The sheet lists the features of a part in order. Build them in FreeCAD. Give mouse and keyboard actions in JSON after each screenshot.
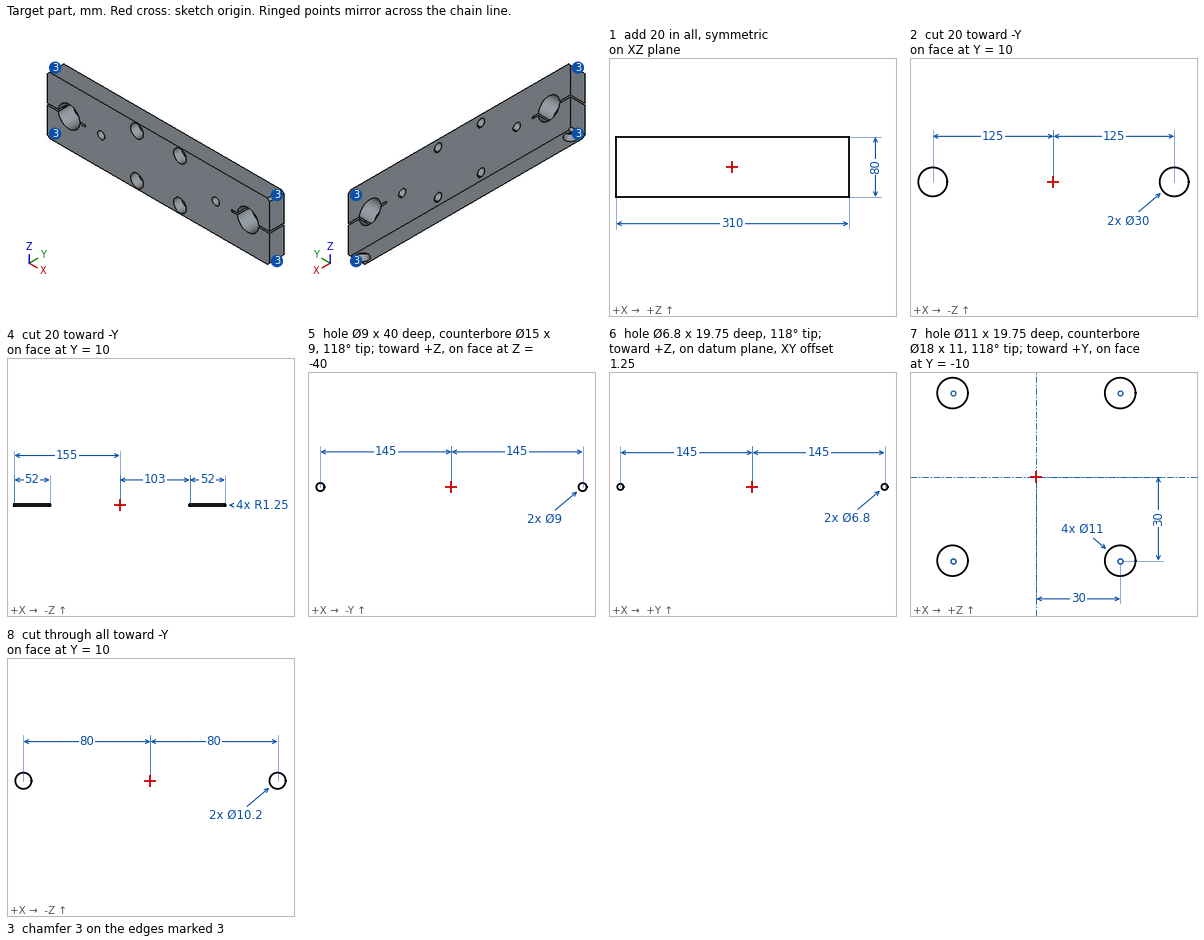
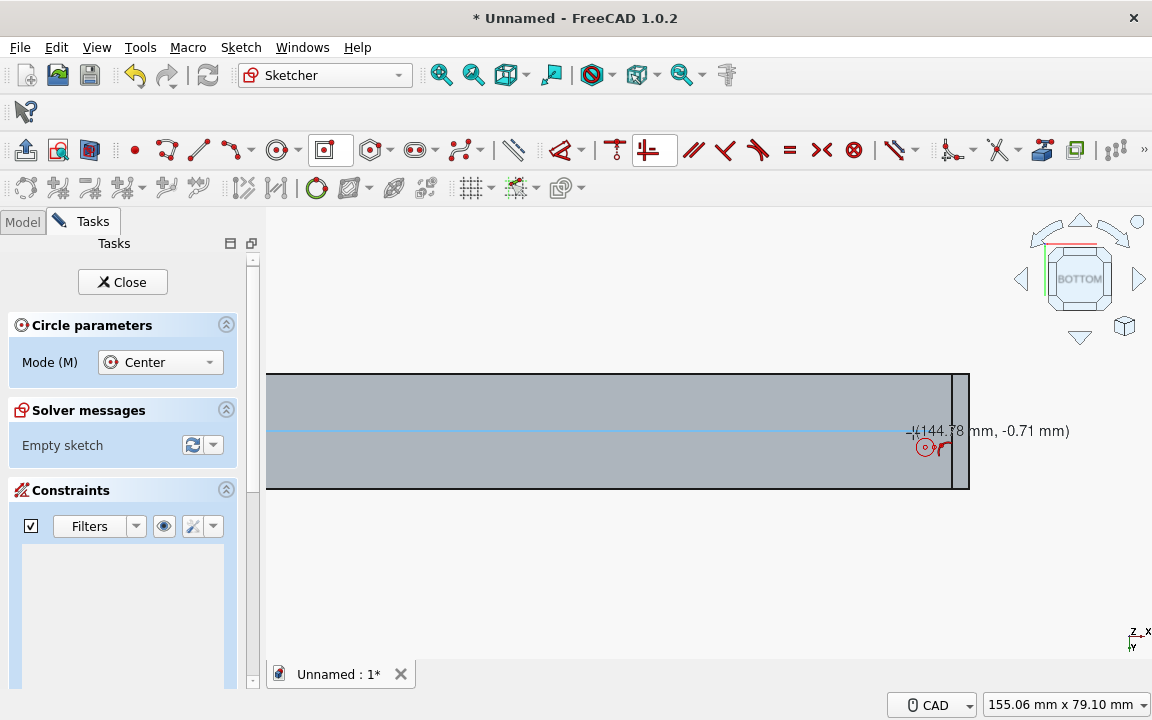
{"action": "scroll", "coordinate": [881, 434], "scroll_direction": "down", "scroll_amount": 6}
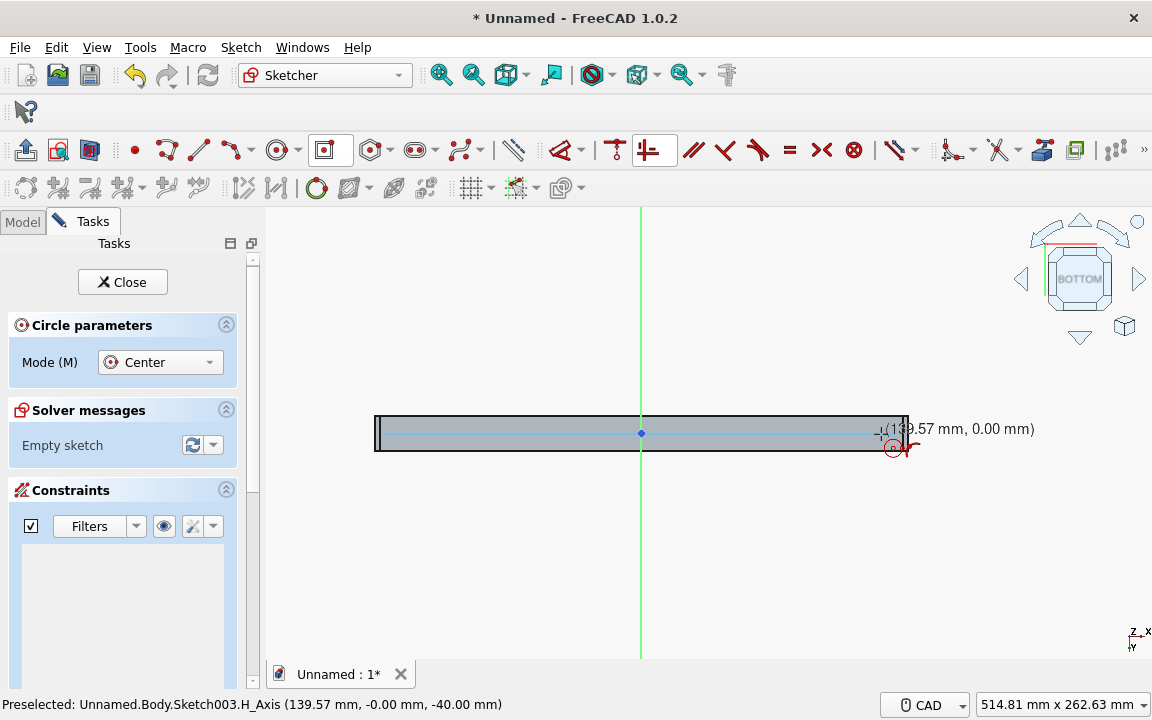
{"action": "left_click", "coordinate": [891, 434]}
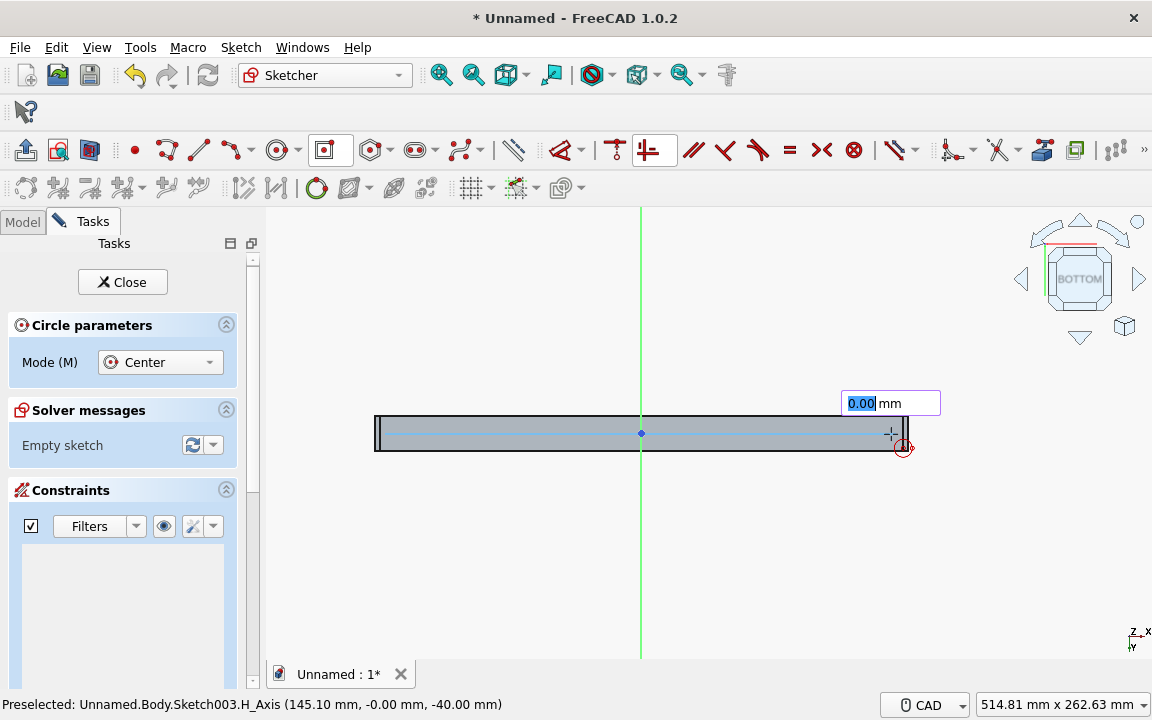
{"action": "scroll", "coordinate": [888, 441], "scroll_direction": "up", "scroll_amount": 4}
{"action": "mouse_move", "coordinate": [888, 440]}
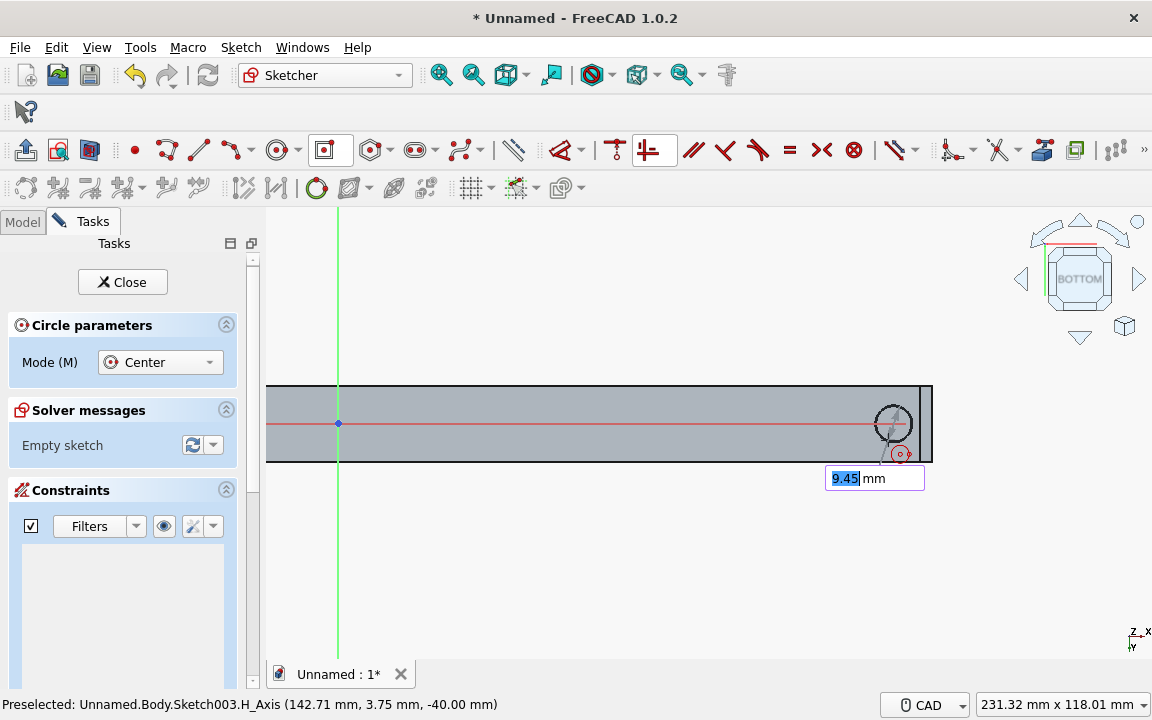
{"action": "type", "text": "9"}
{"action": "key", "text": "Return"}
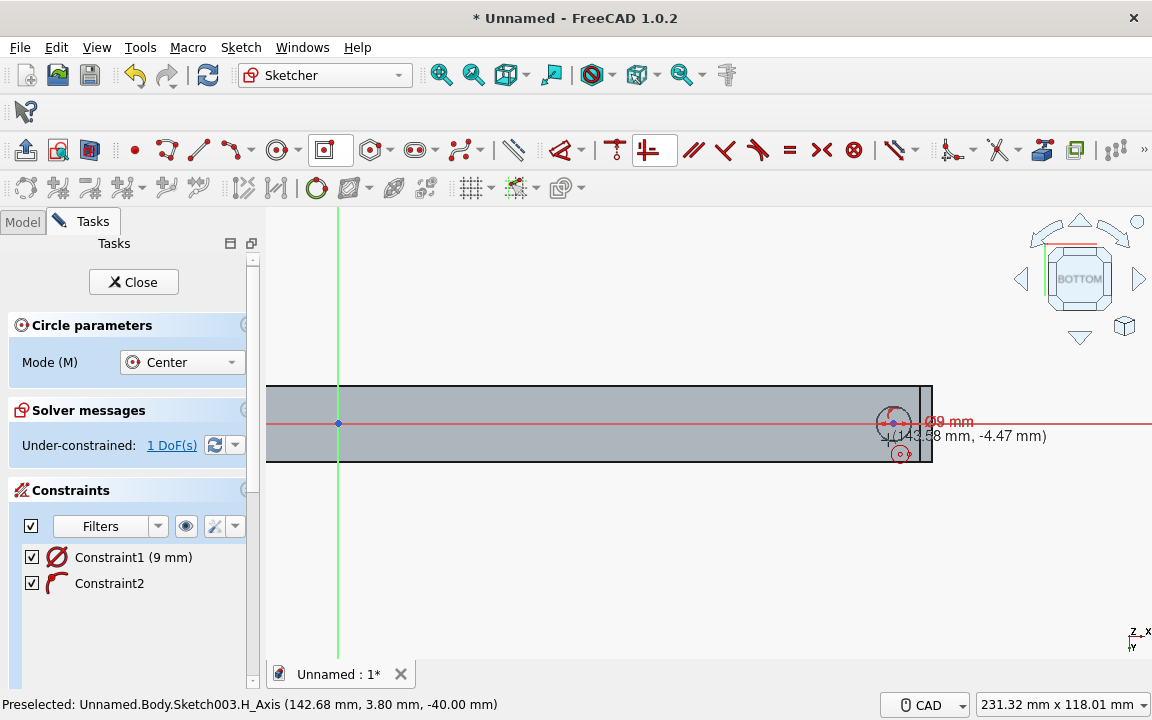
{"action": "scroll", "coordinate": [887, 440], "scroll_direction": "down", "scroll_amount": 4}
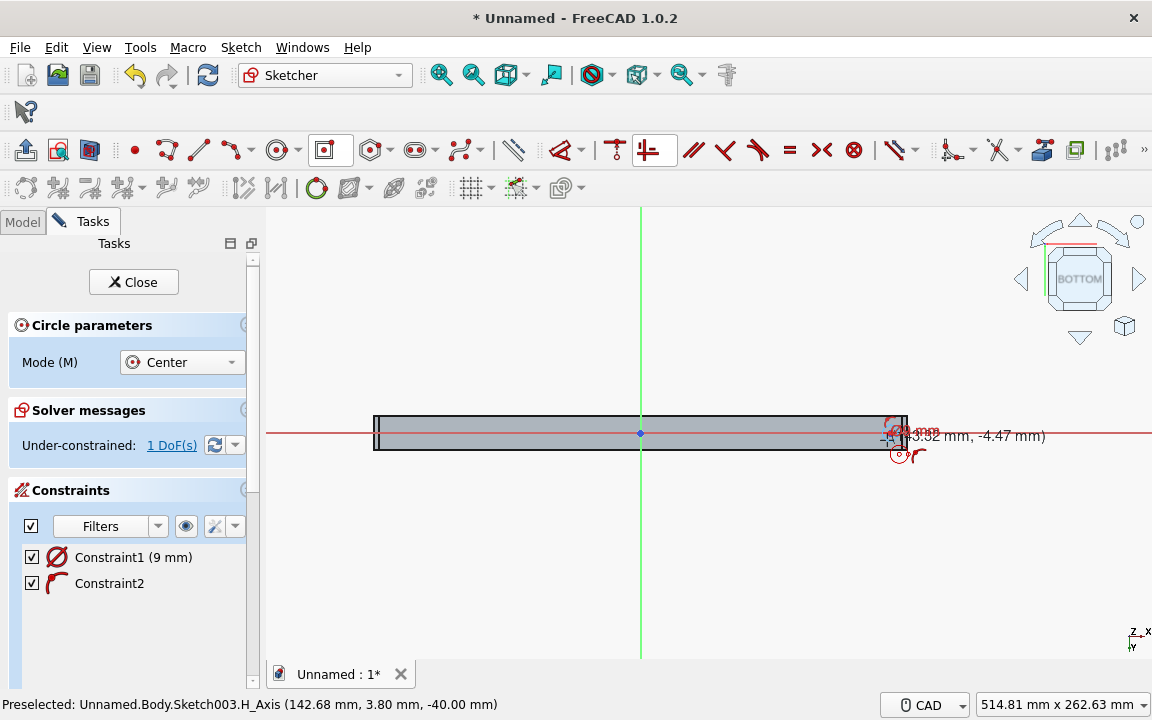
{"action": "scroll", "coordinate": [391, 433], "scroll_direction": "up", "scroll_amount": 6}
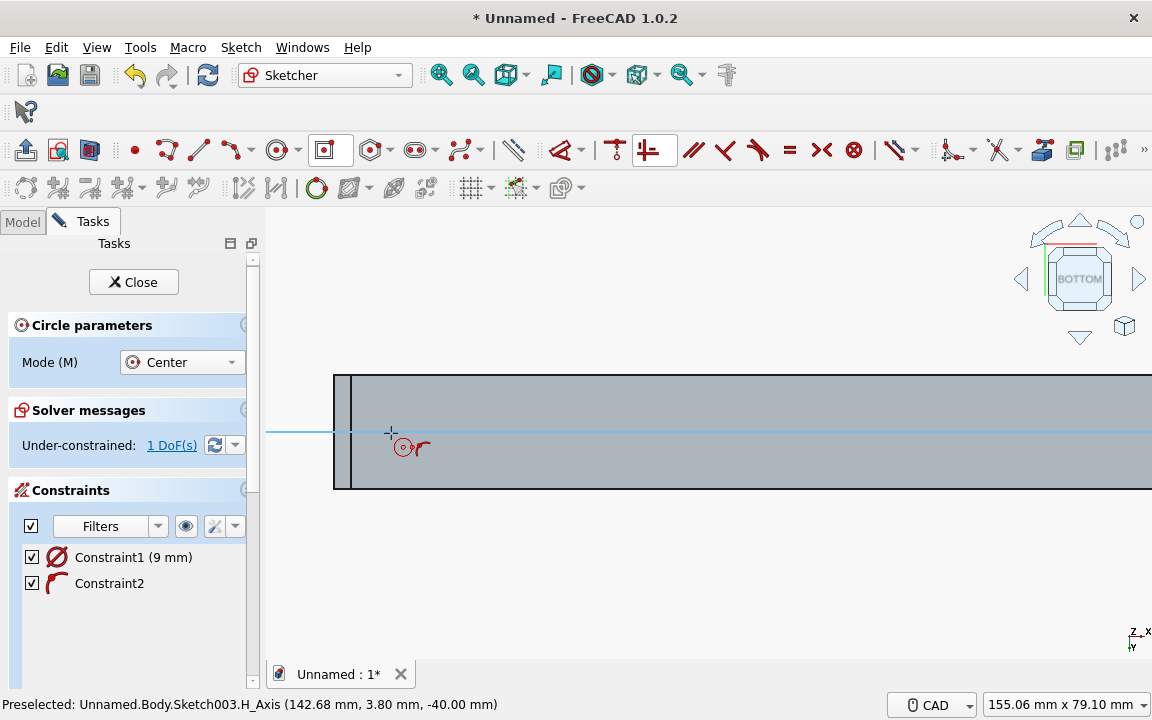
{"action": "scroll", "coordinate": [391, 433], "scroll_direction": "down", "scroll_amount": 6}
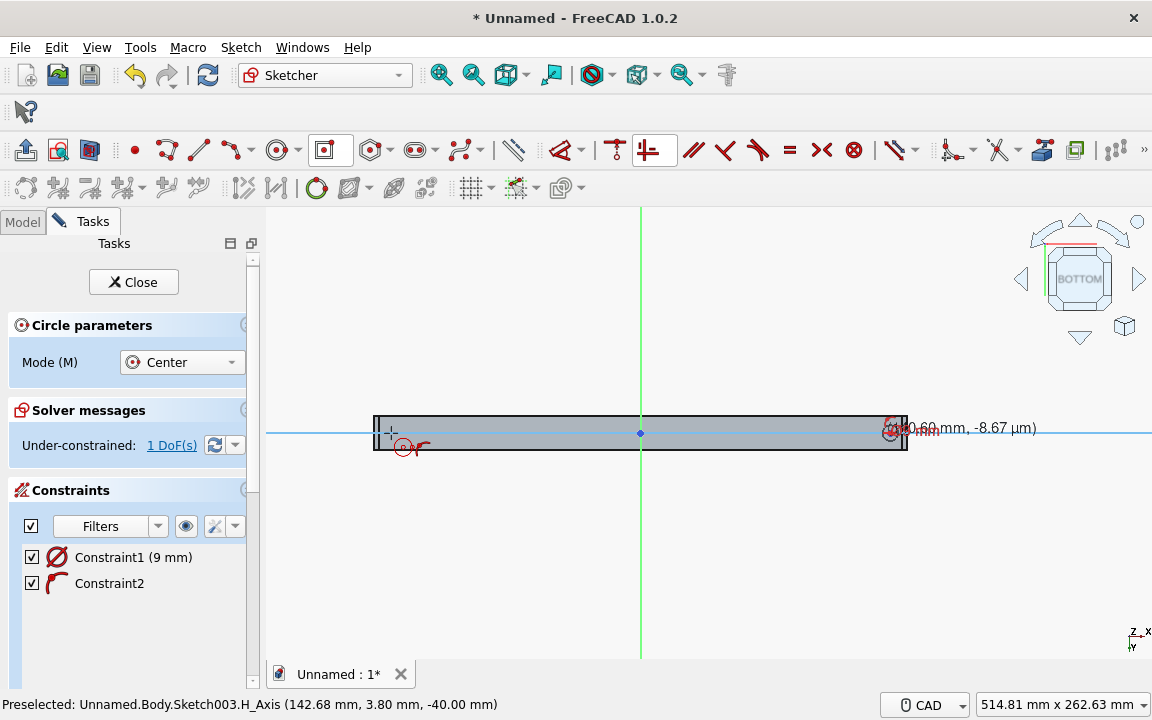
{"action": "left_click", "coordinate": [391, 433]}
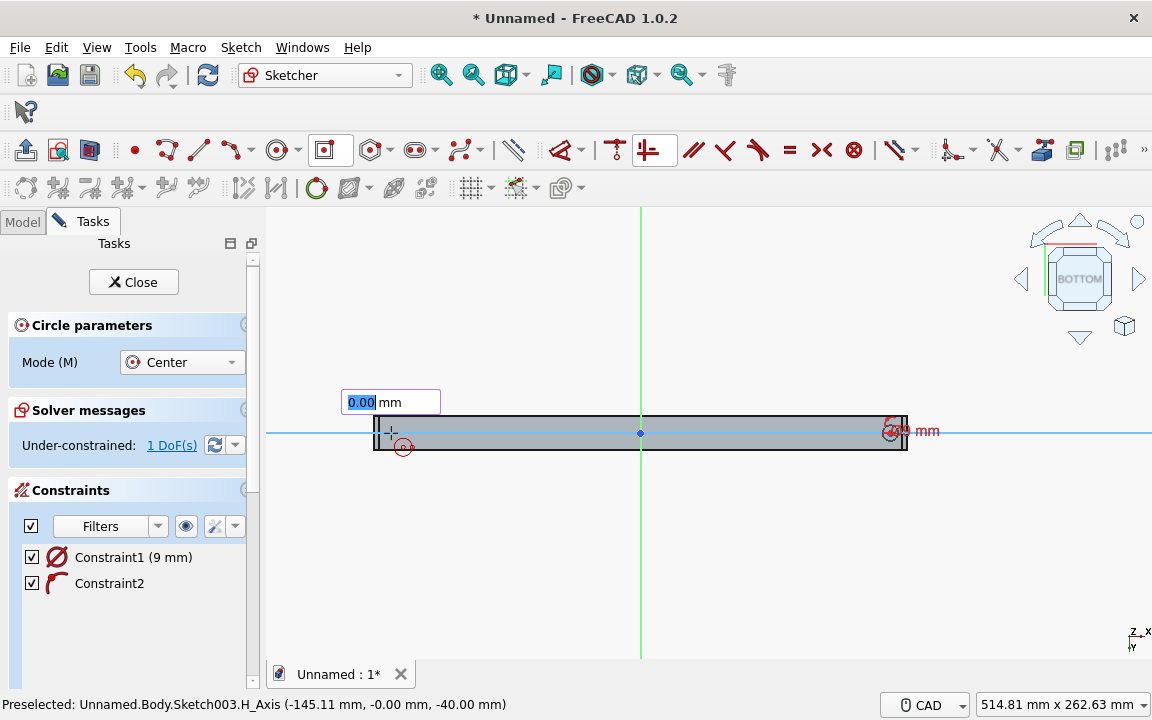
{"action": "scroll", "coordinate": [389, 440], "scroll_direction": "up", "scroll_amount": 4}
{"action": "mouse_move", "coordinate": [388, 440]}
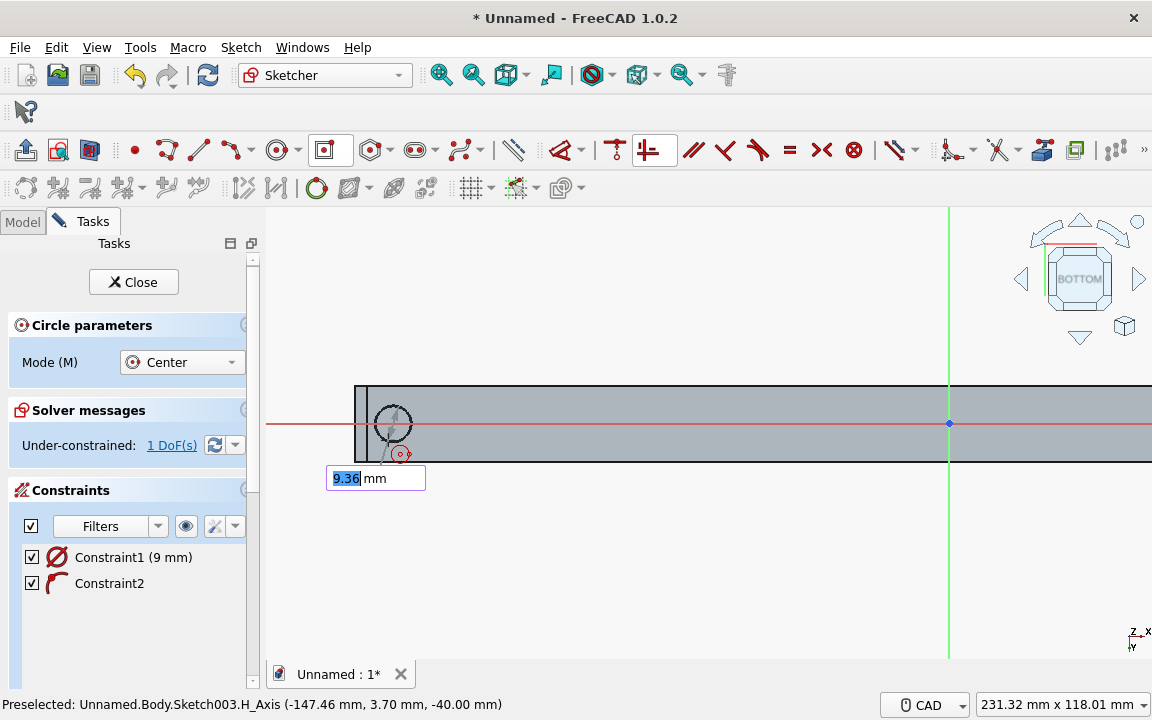
{"action": "type", "text": "9"}
{"action": "key", "text": "Return"}
{"action": "key", "text": "Escape"}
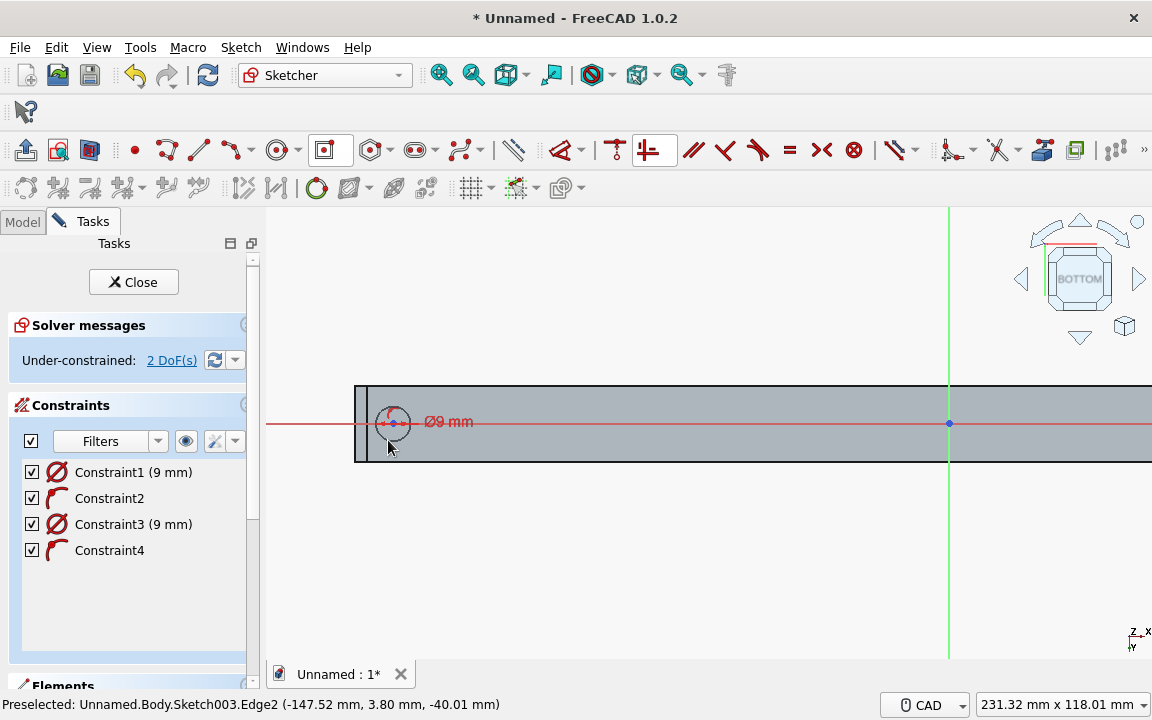
{"action": "left_click", "coordinate": [560, 150]}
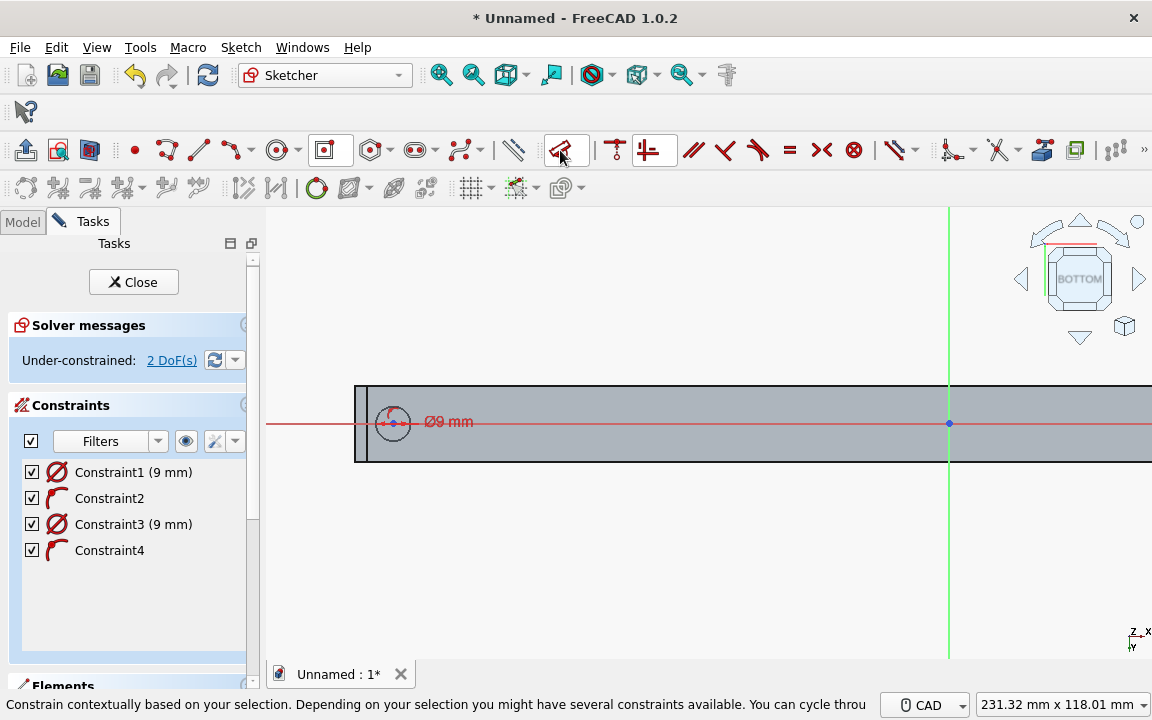
{"action": "scroll", "coordinate": [389, 440], "scroll_direction": "down", "scroll_amount": 4}